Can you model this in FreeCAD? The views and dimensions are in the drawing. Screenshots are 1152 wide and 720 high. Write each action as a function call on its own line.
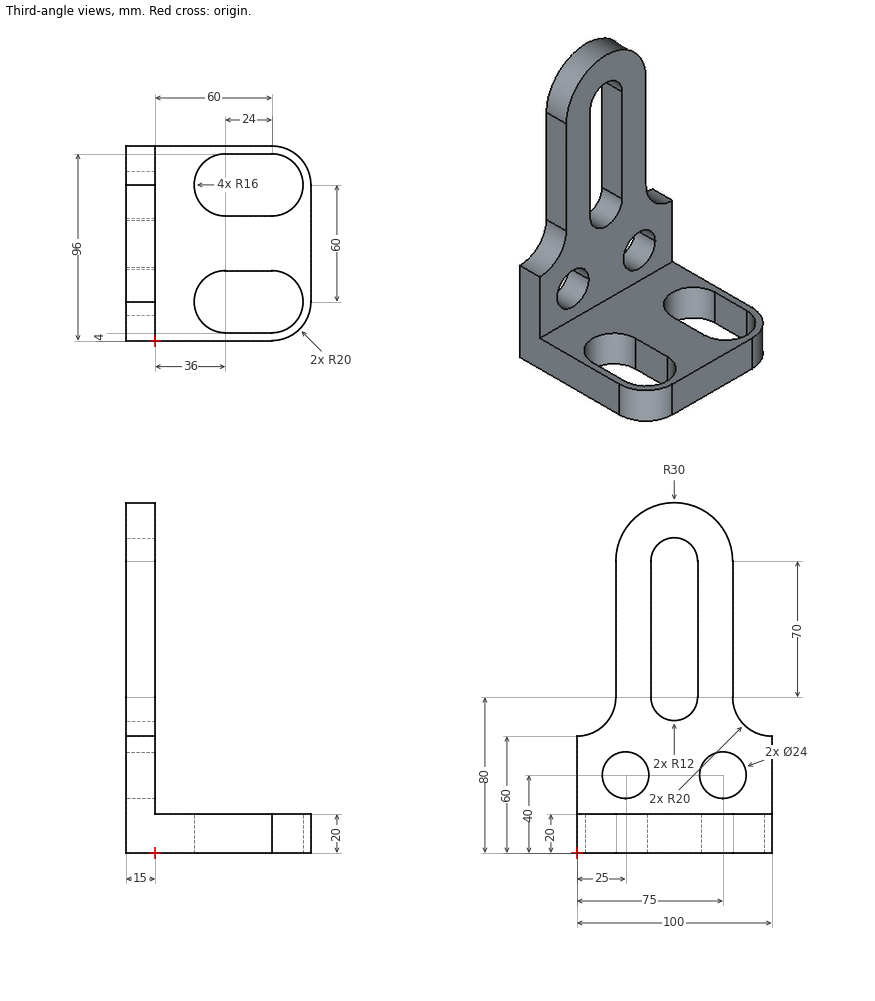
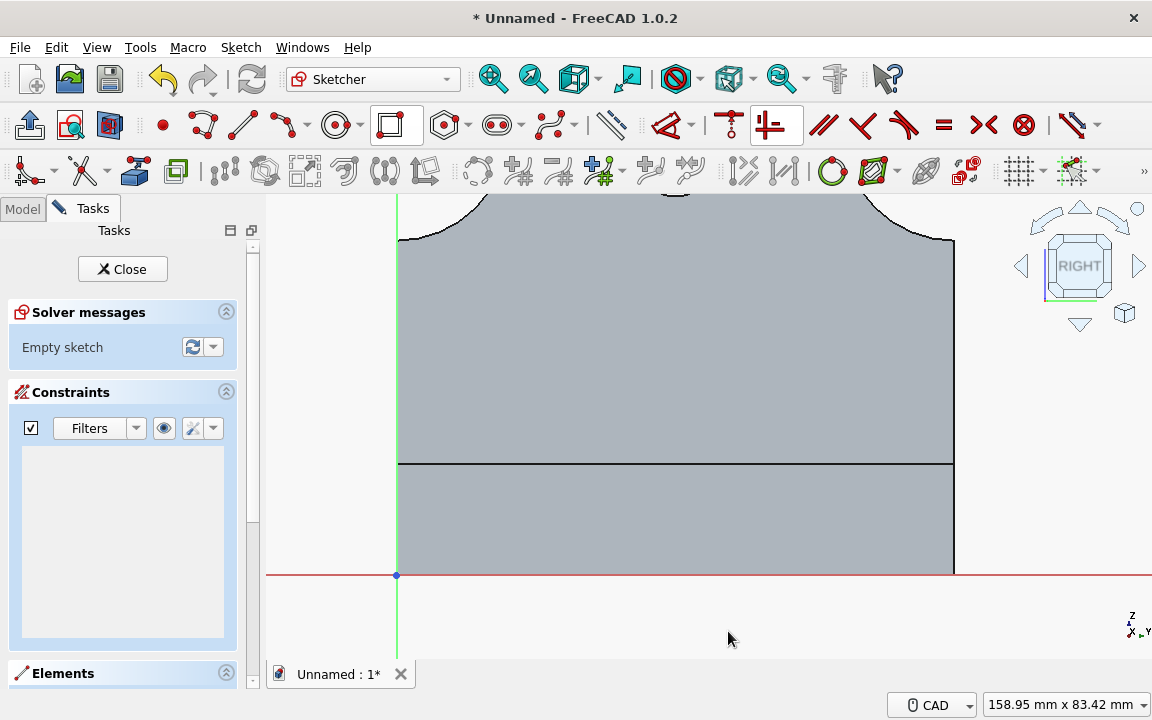
click(336, 126)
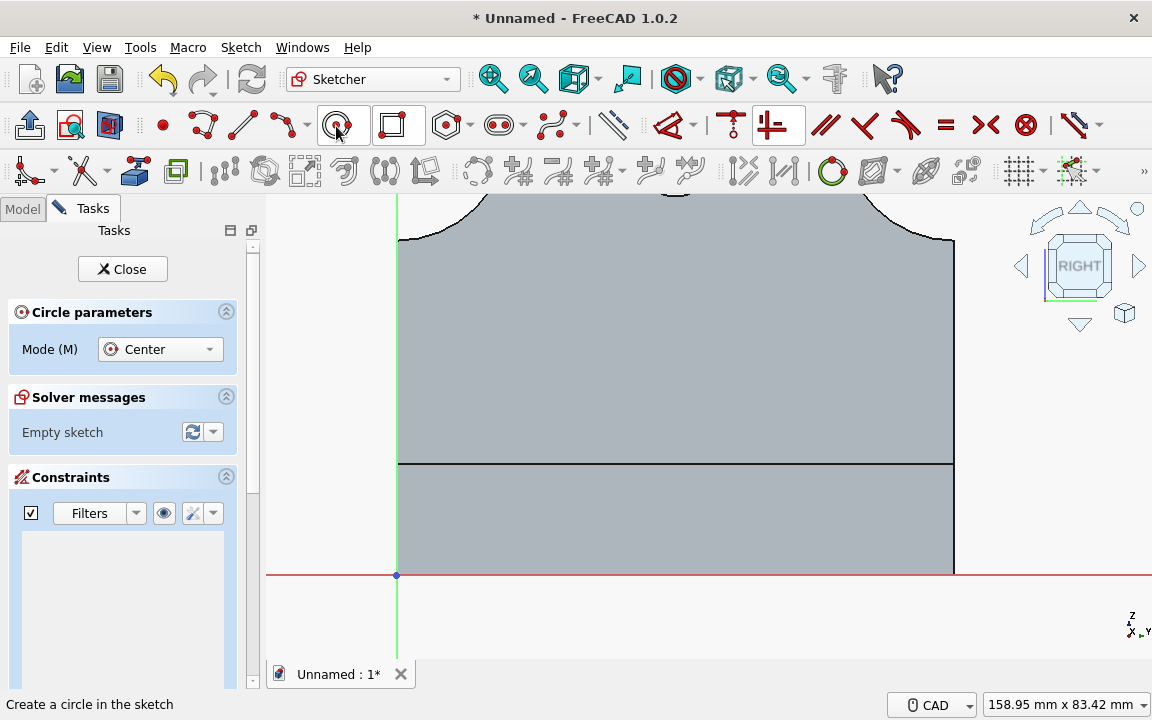
click(815, 352)
move(862, 305)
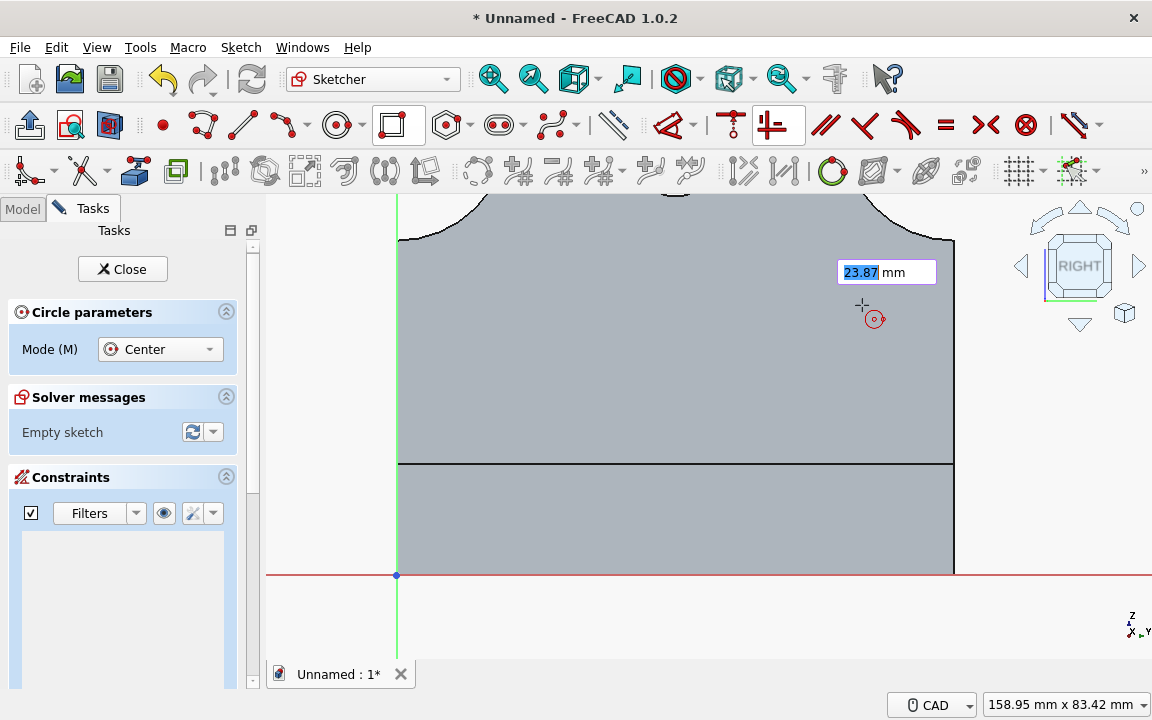
text(24)
key(Return)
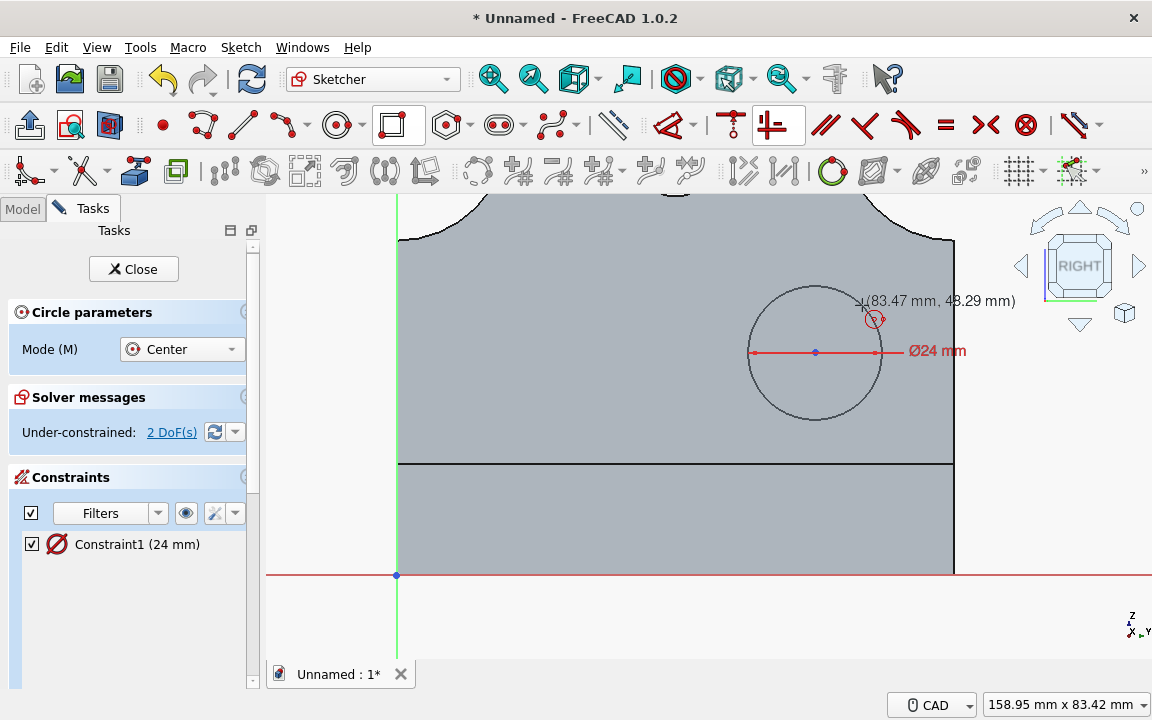
click(536, 352)
move(583, 305)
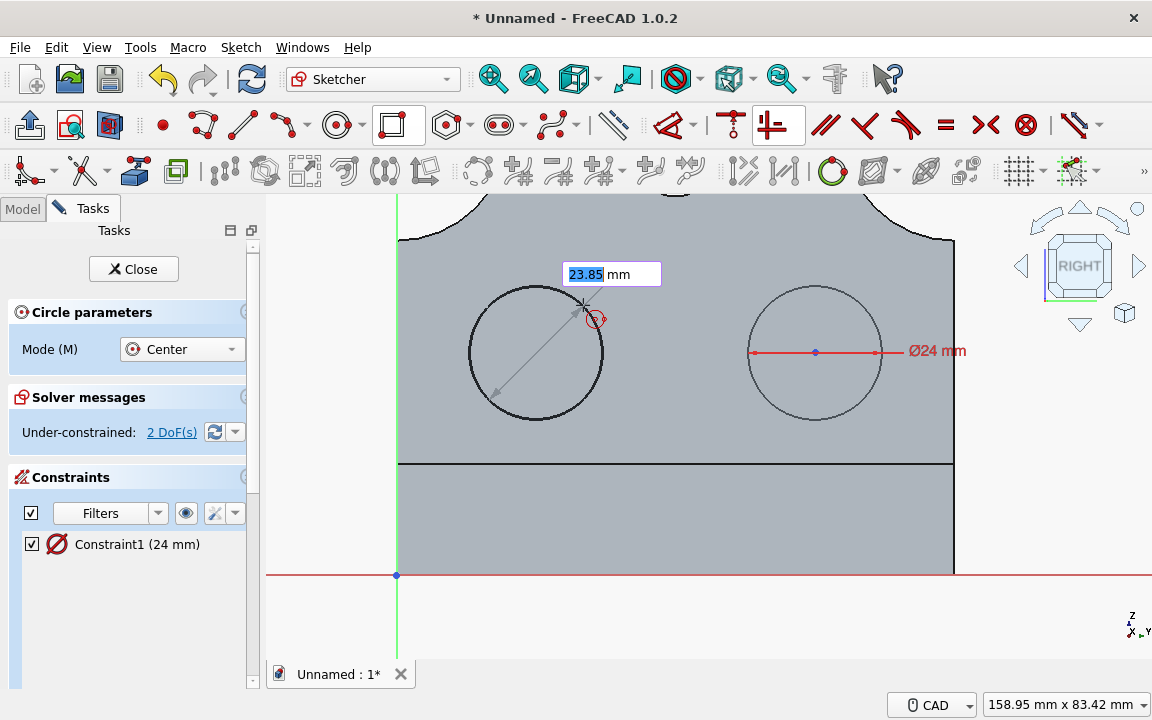
text(24)
key(Return)
key(Escape)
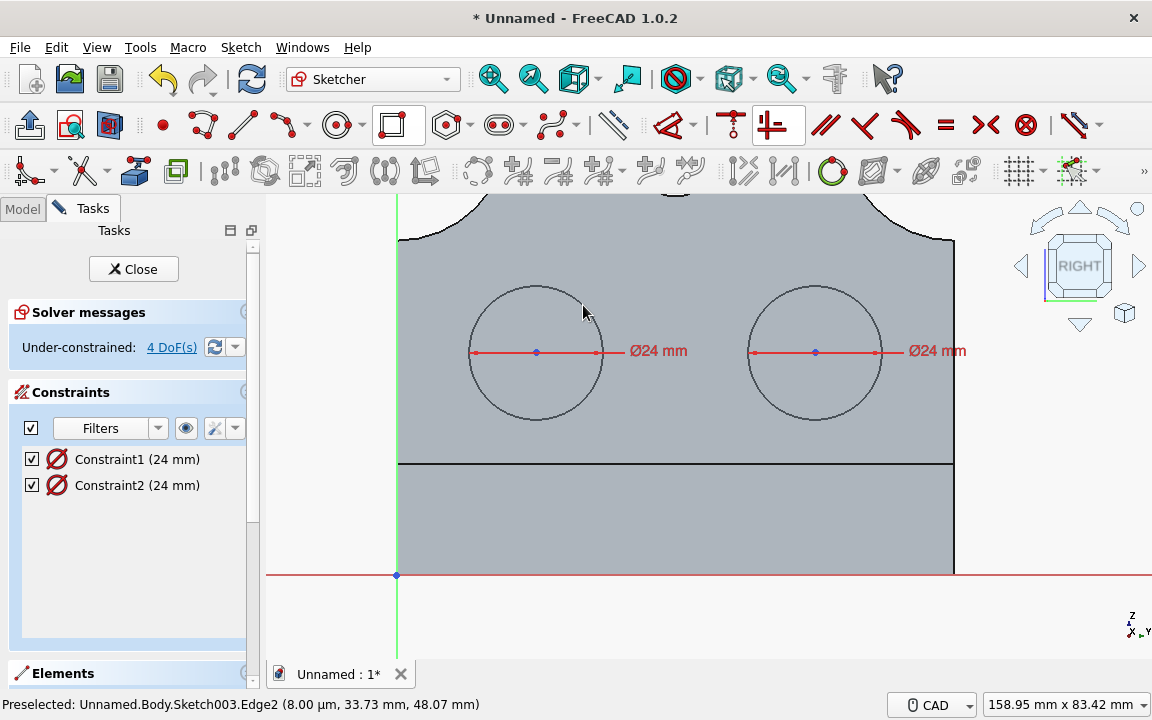
key(d)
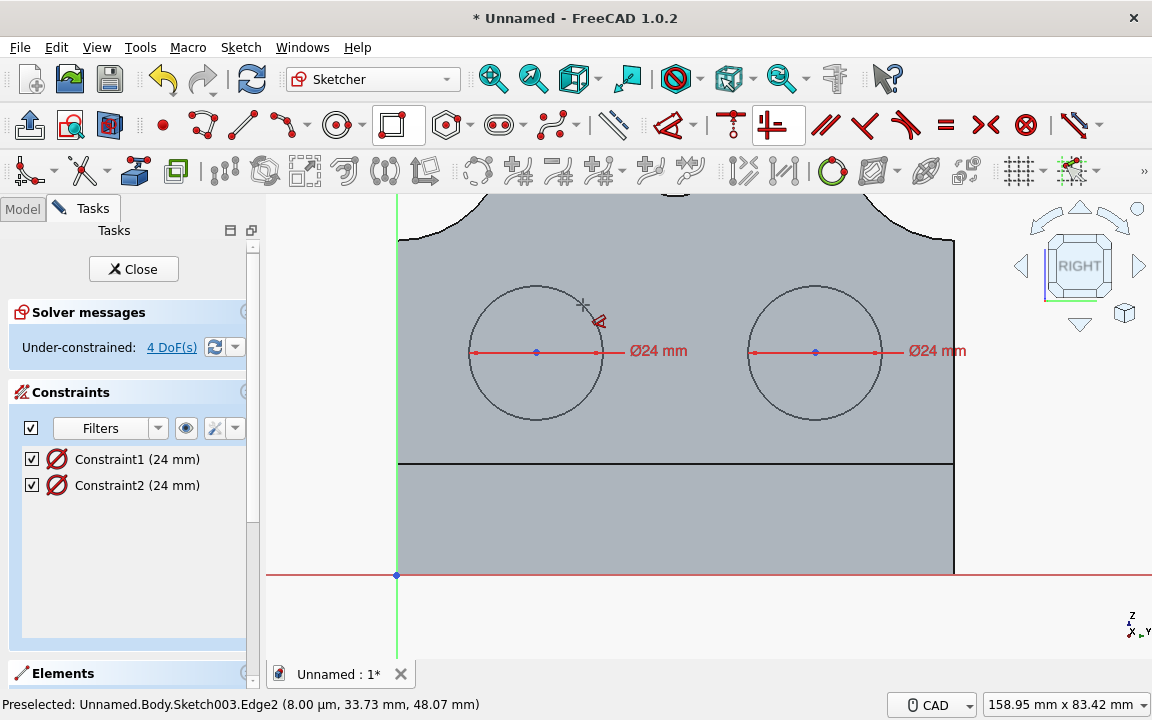
click(815, 353)
click(606, 609)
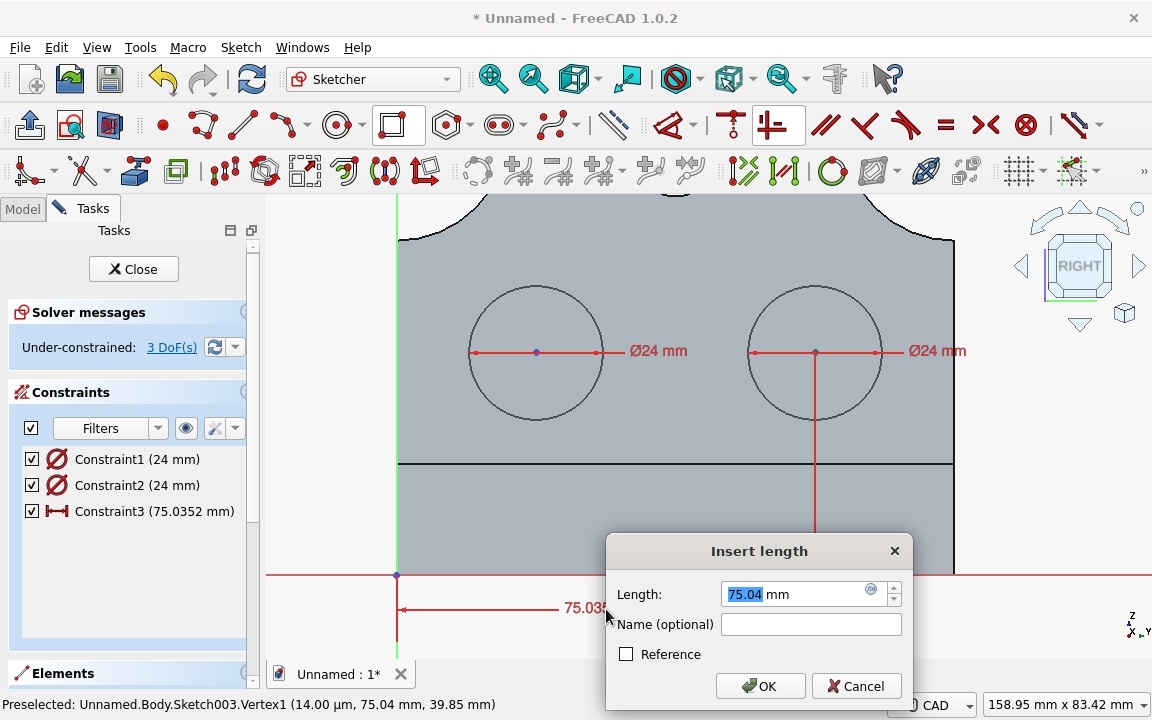
text(75)
key(Return)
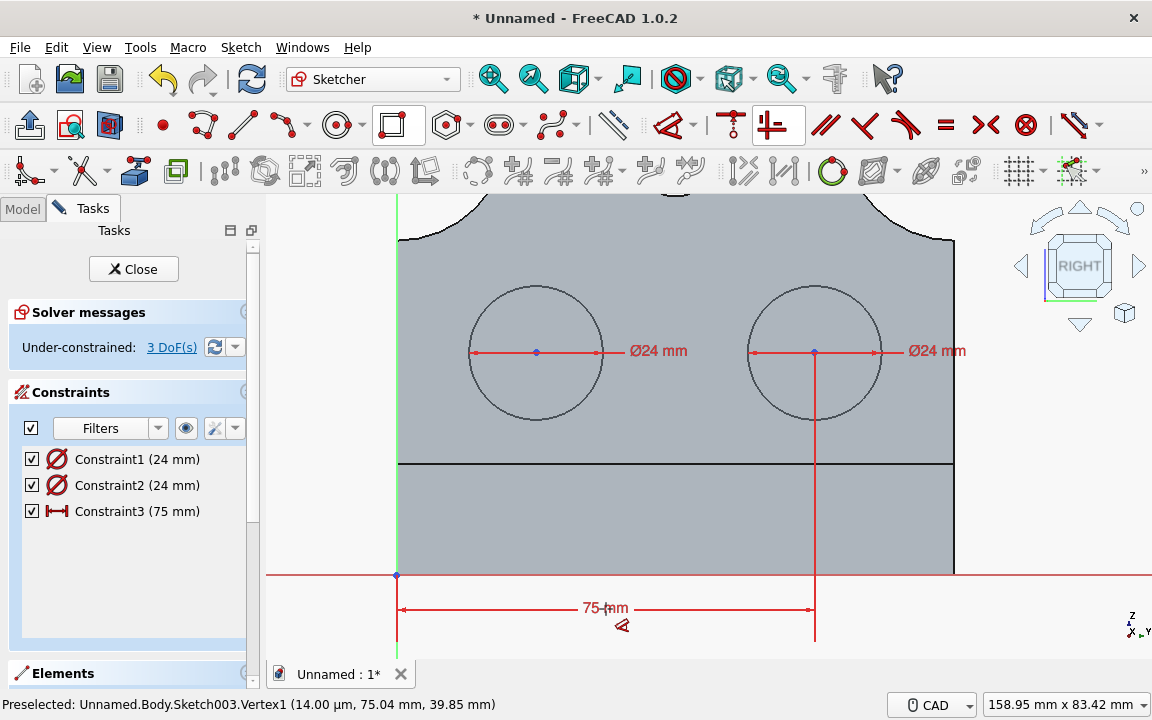
click(815, 353)
click(363, 464)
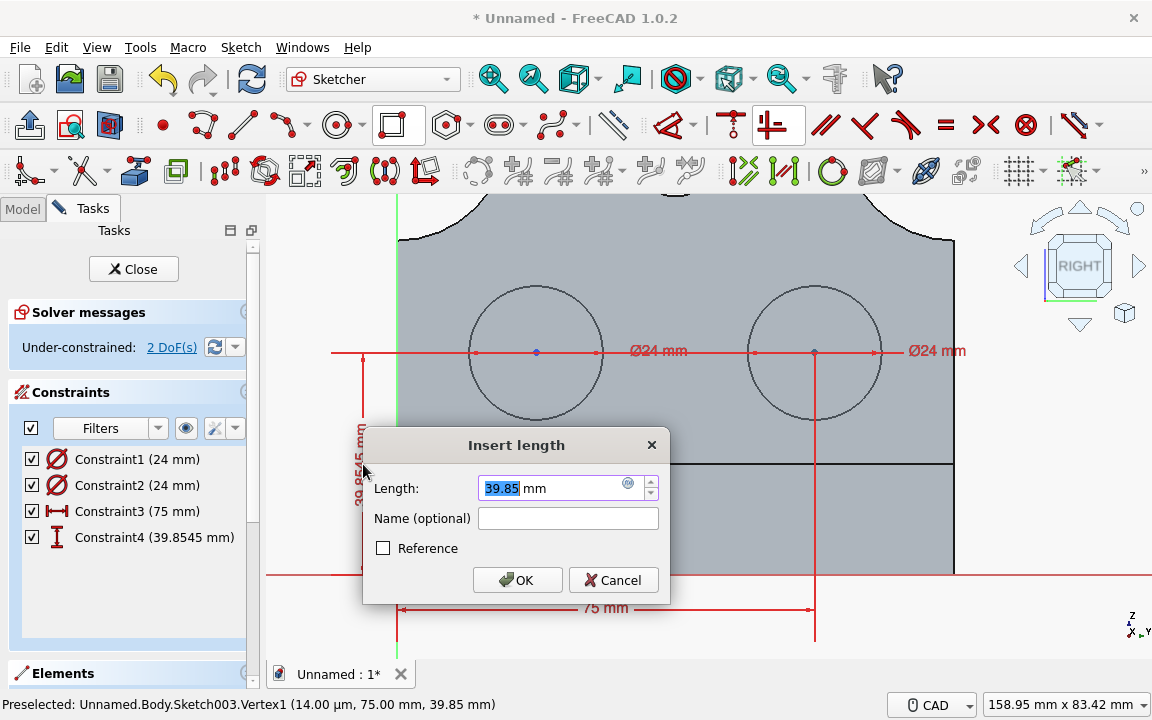
text(40)
key(Return)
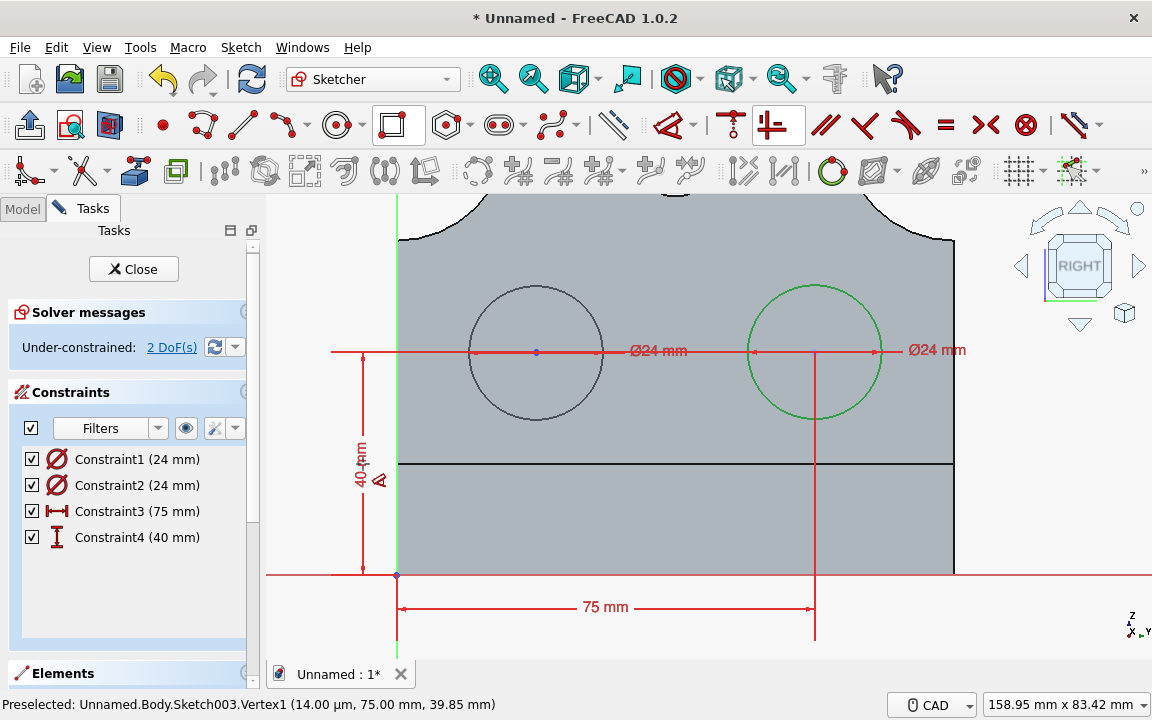
click(536, 353)
click(466, 609)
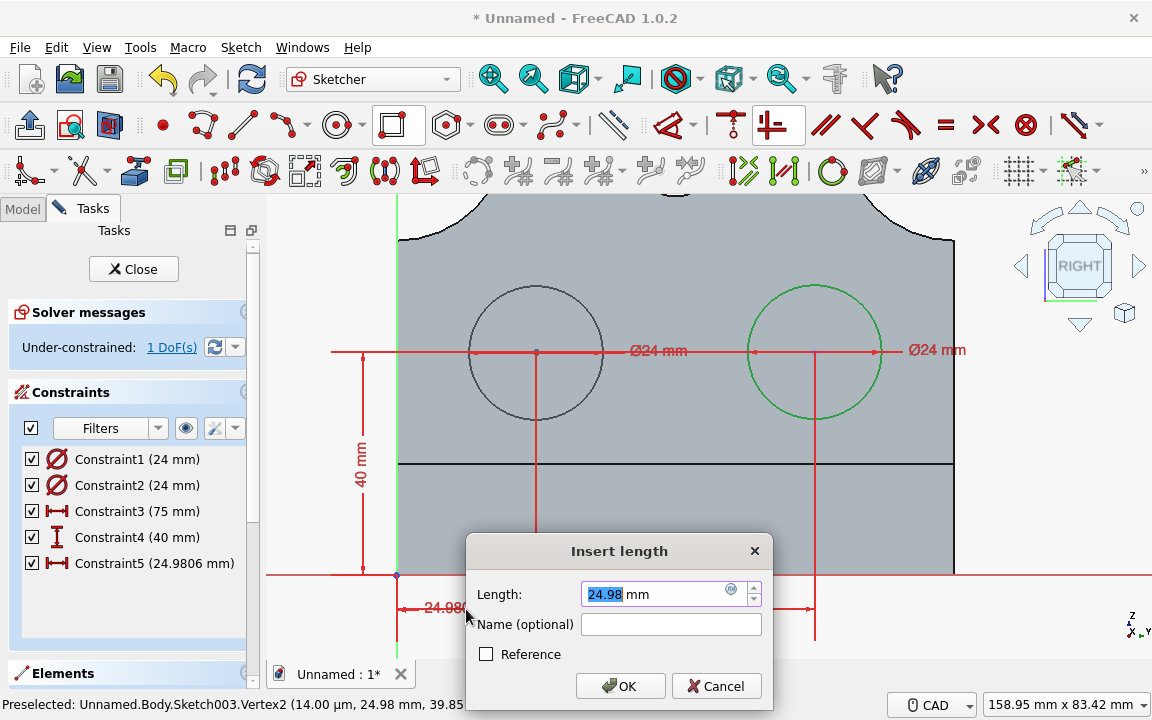
text(25)
key(Return)